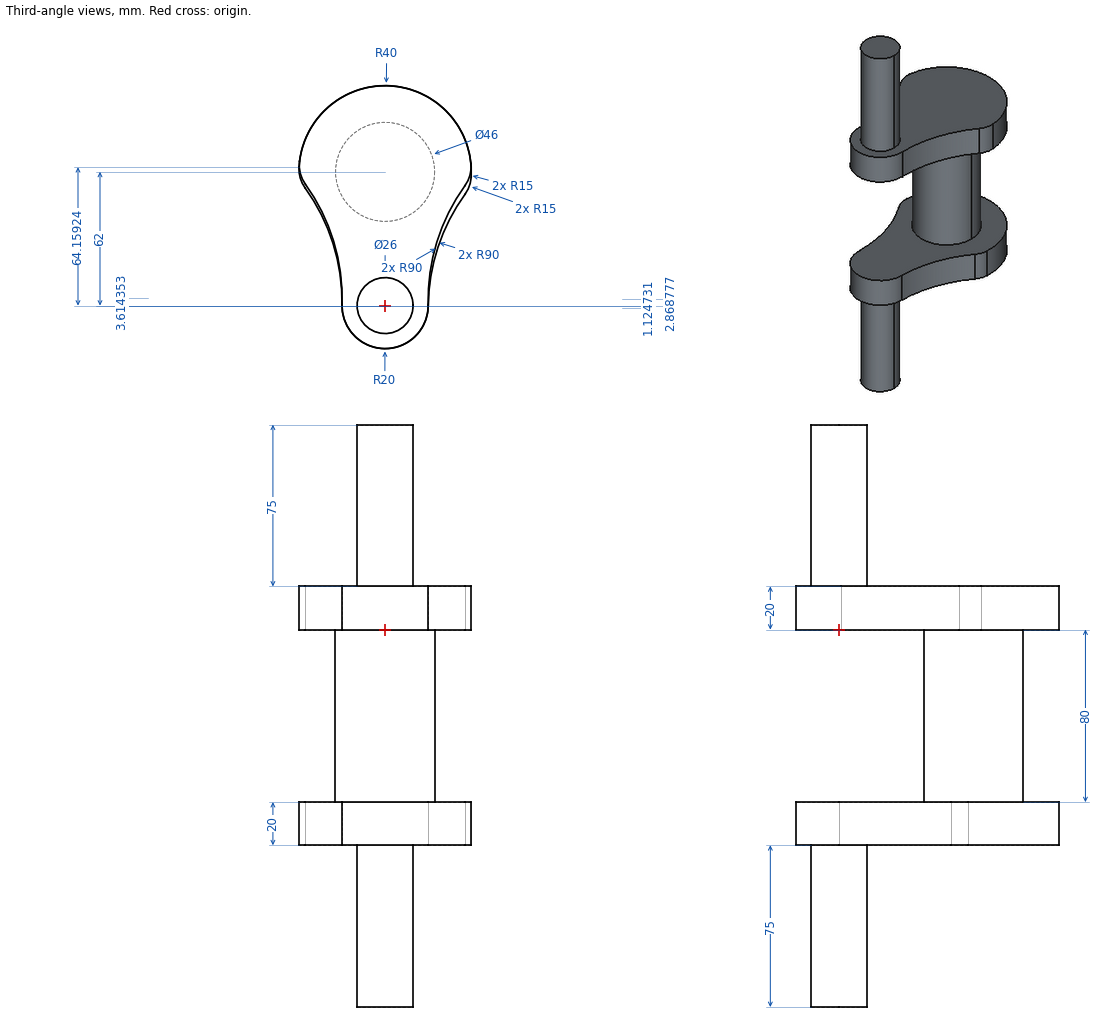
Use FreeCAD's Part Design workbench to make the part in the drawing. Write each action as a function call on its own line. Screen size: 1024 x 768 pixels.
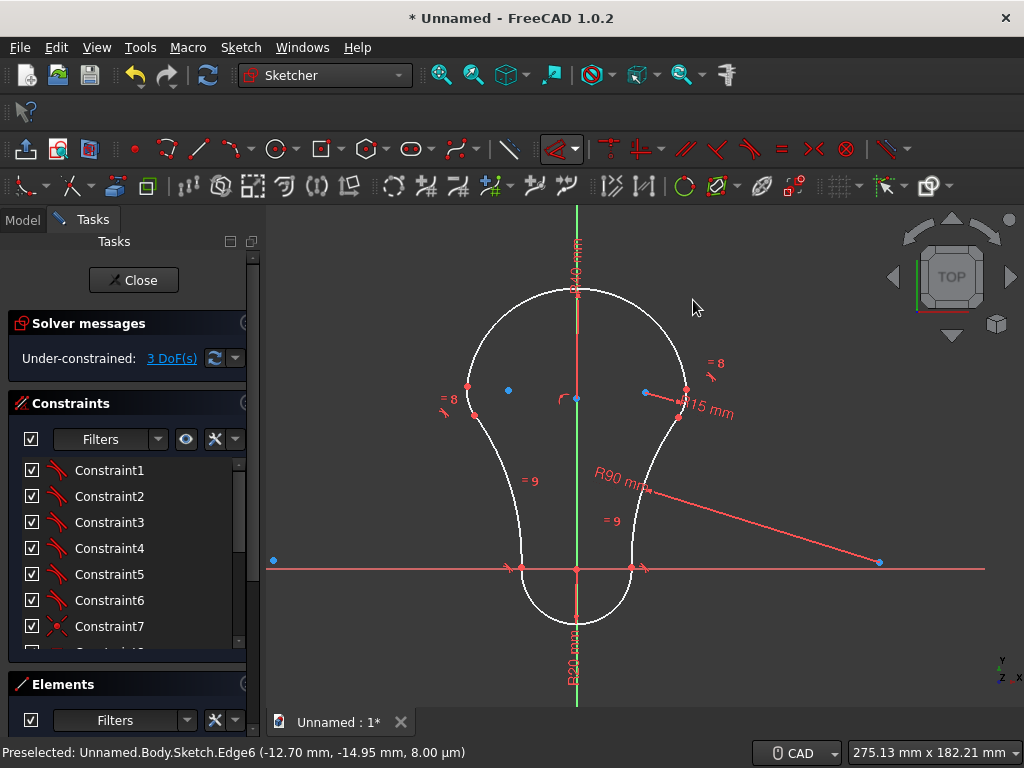
click(577, 399)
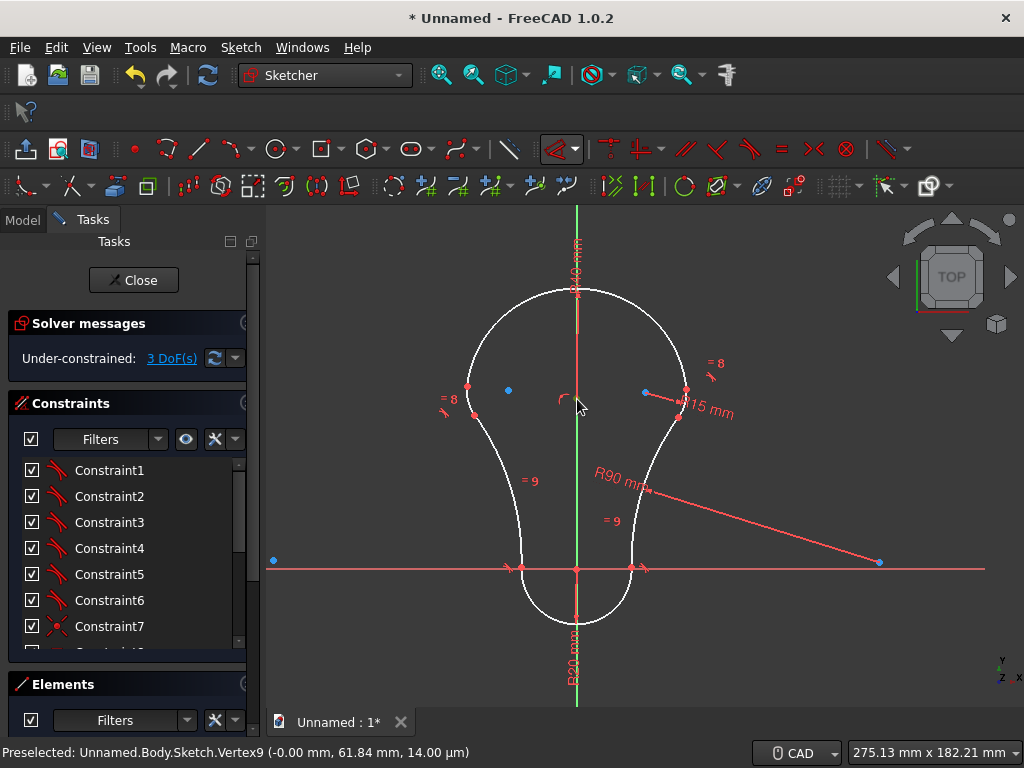
key(i)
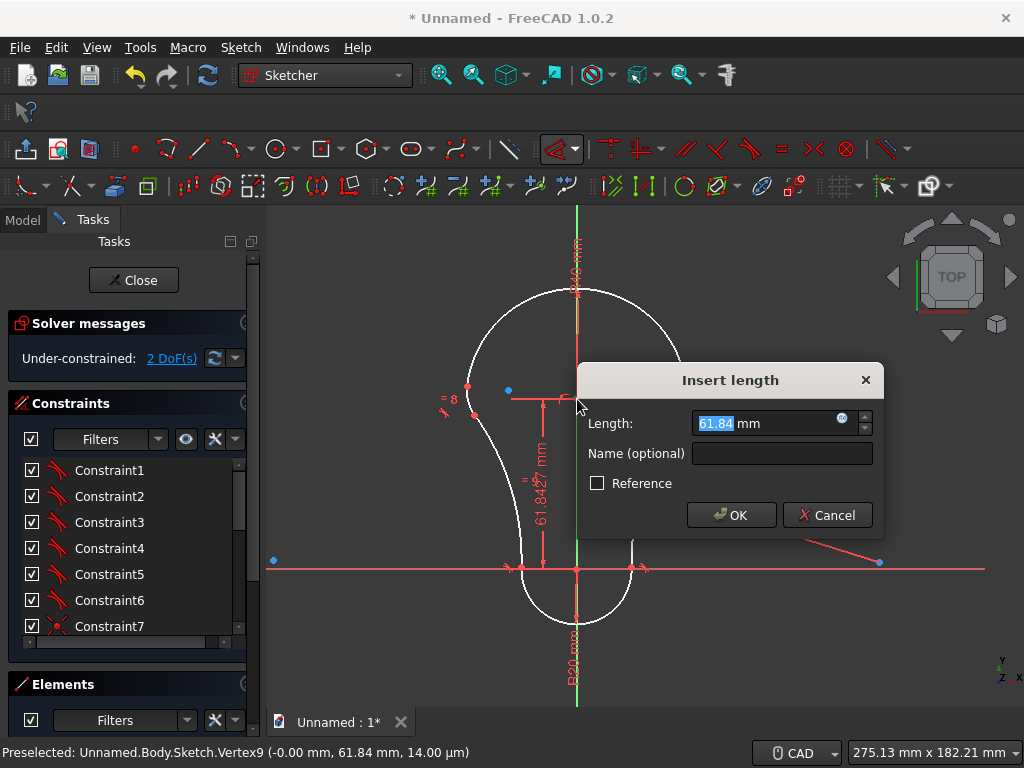
text(62)
key(Return)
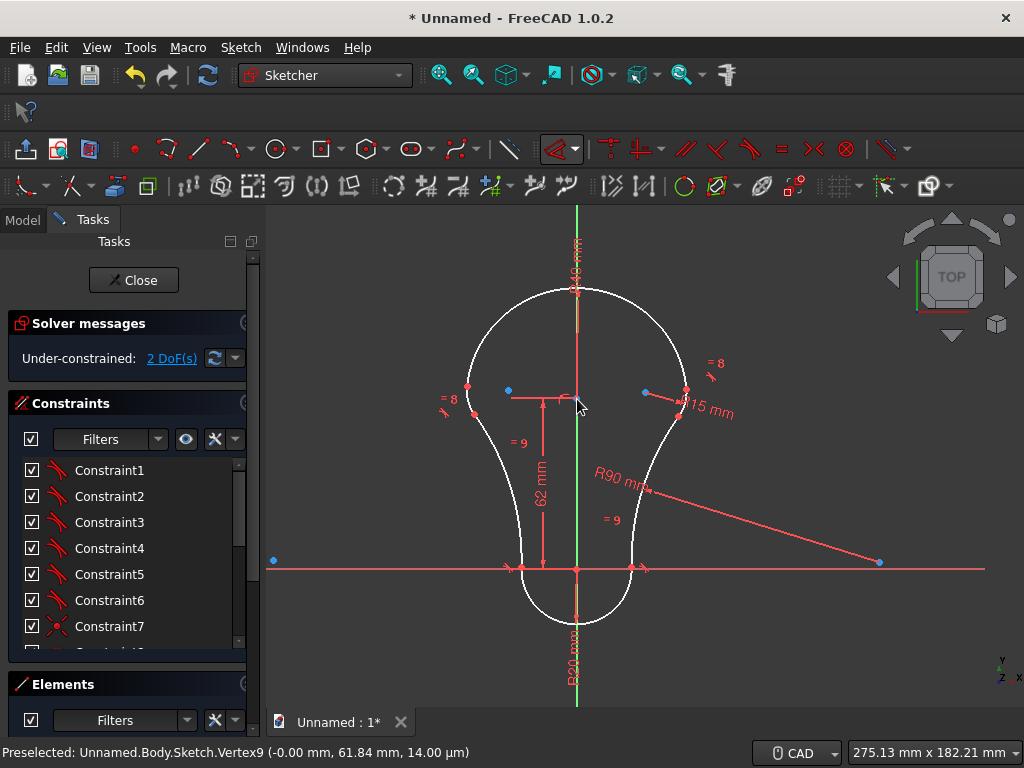
scroll(294, 455, down, 1)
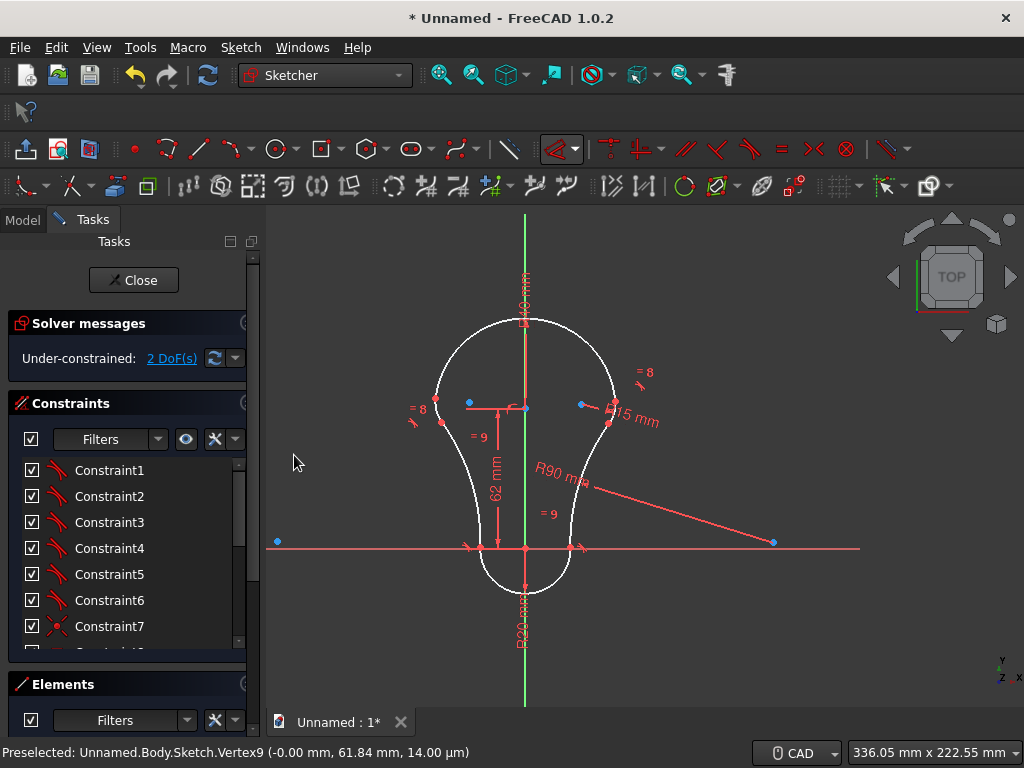
scroll(773, 543, up, 10)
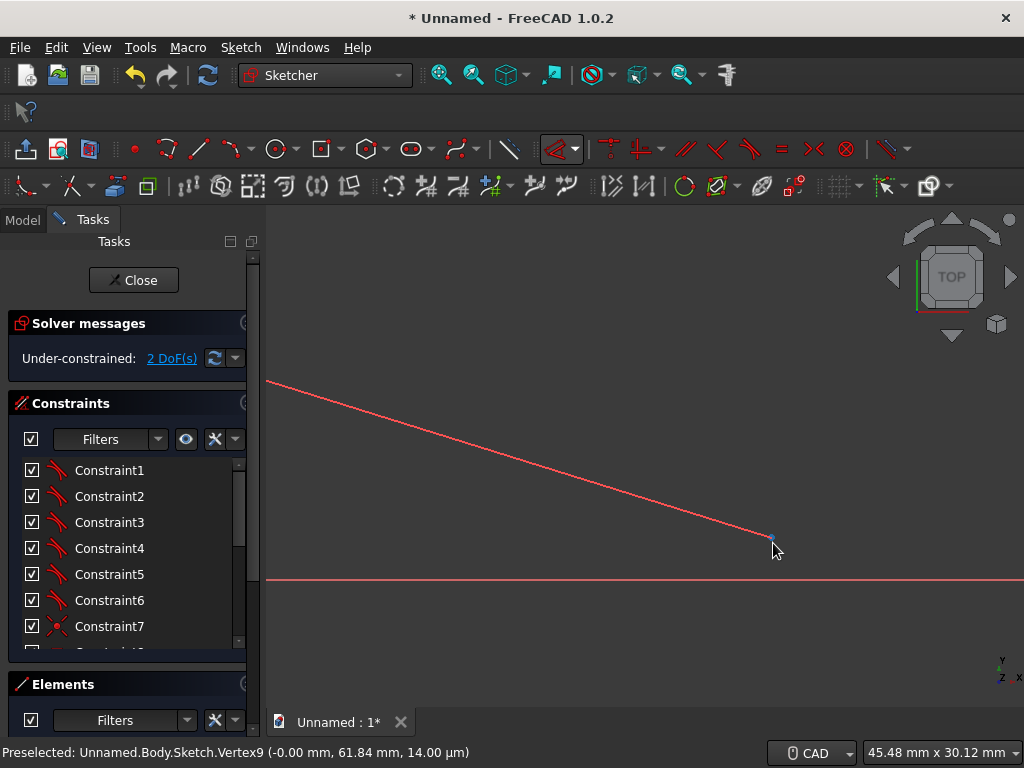
click(772, 538)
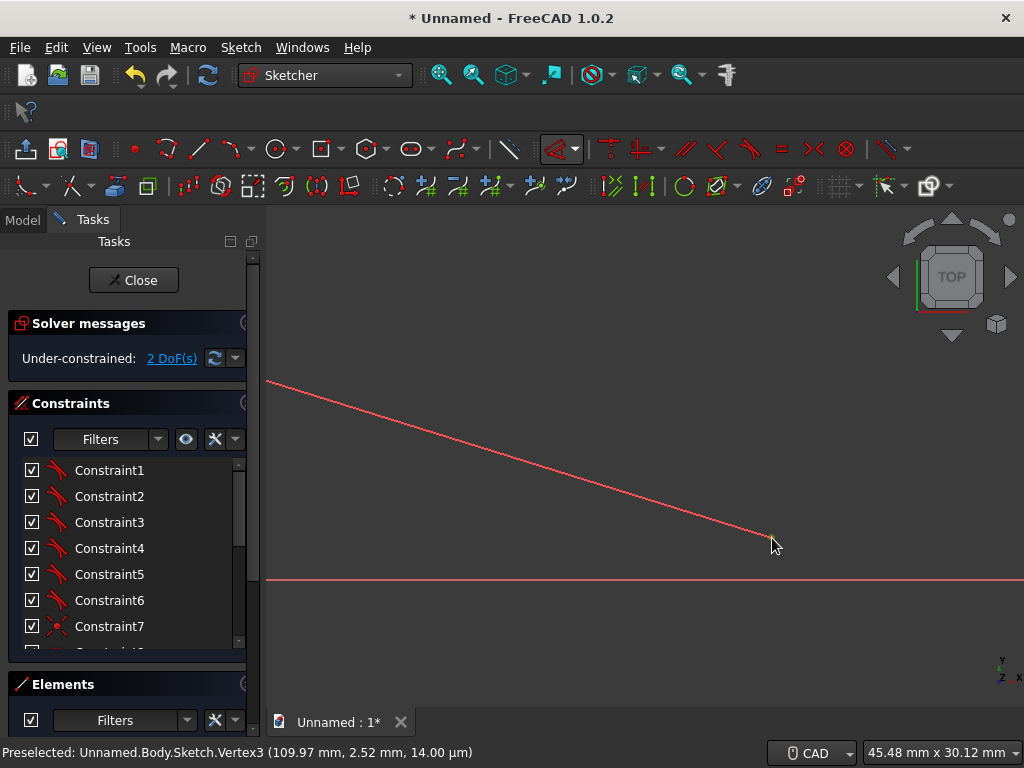
key(i)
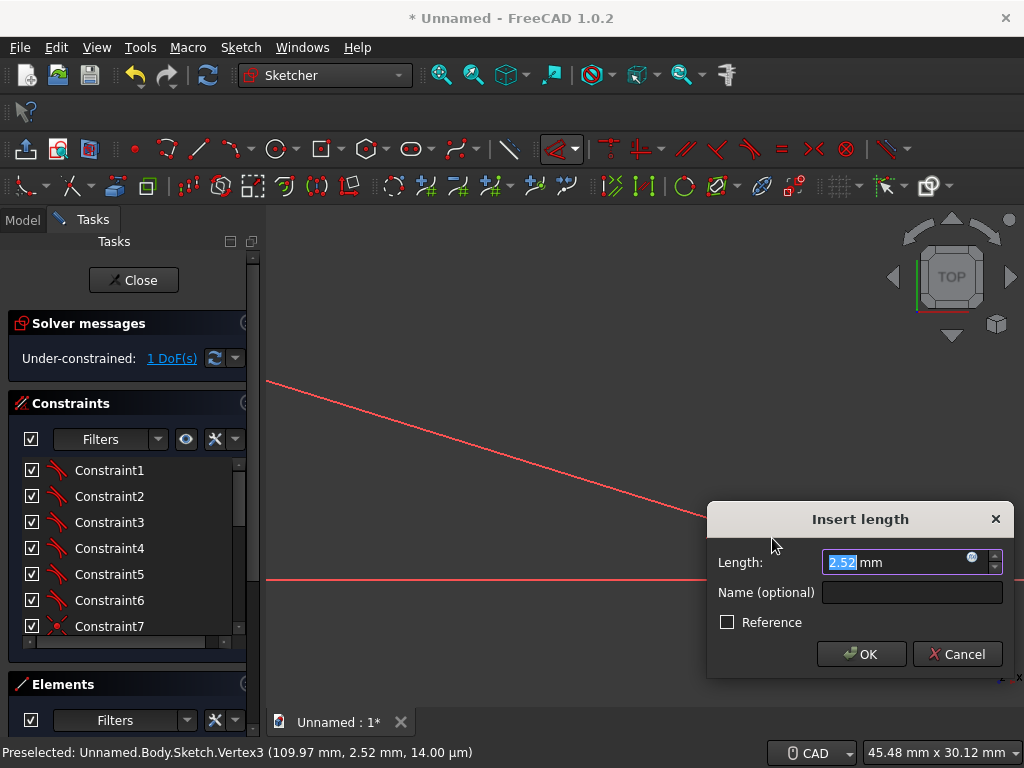
text(2.868777)
key(Return)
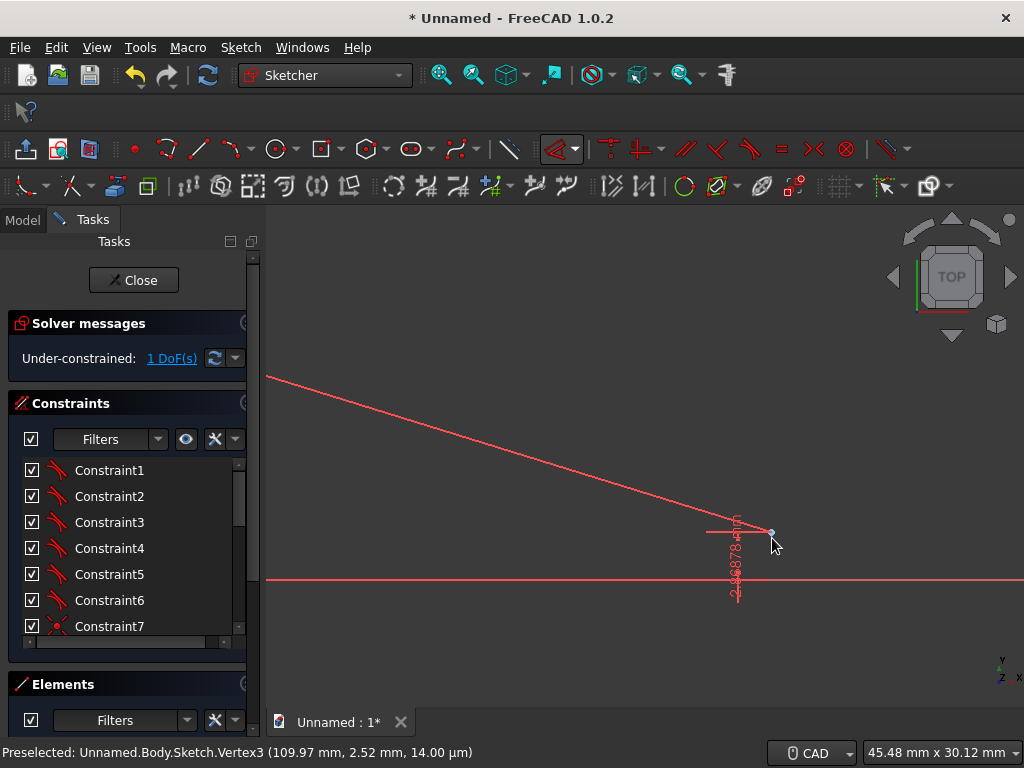
scroll(859, 567, down, 9)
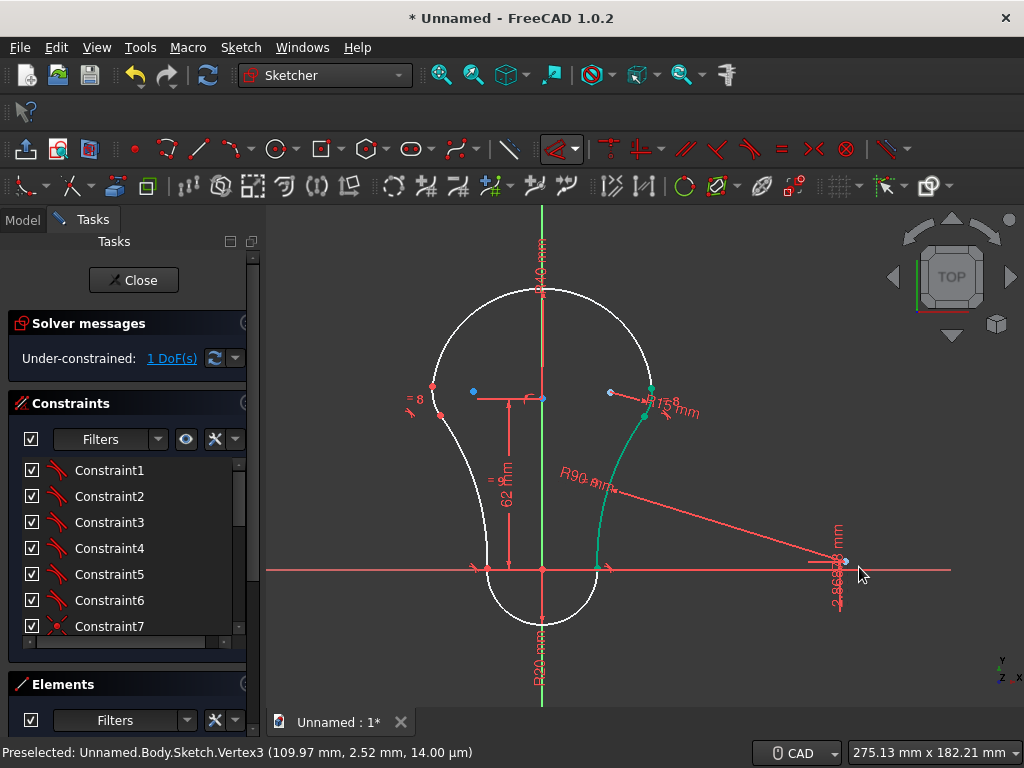
scroll(859, 452, down, 1)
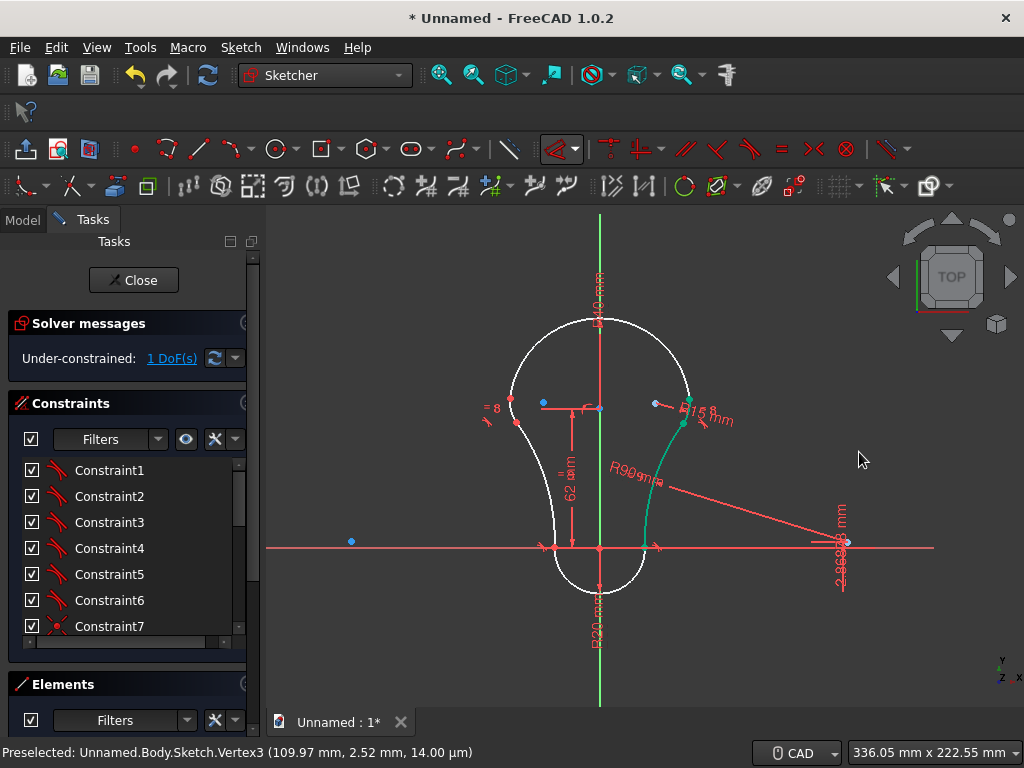
scroll(352, 541, up, 8)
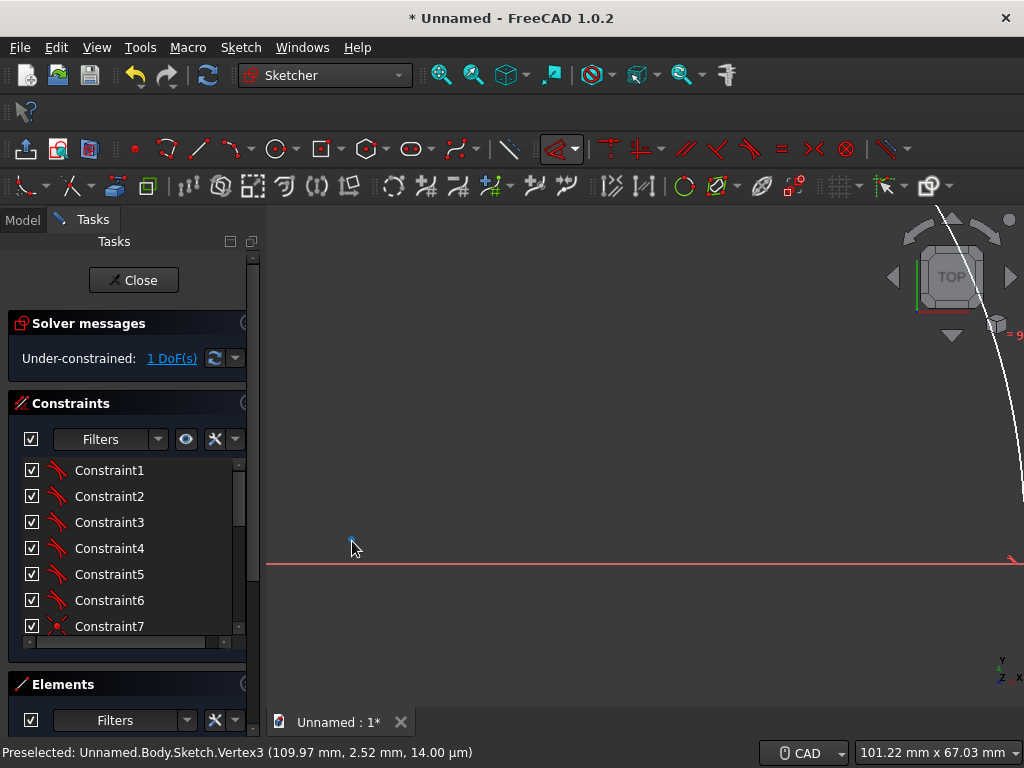
click(351, 538)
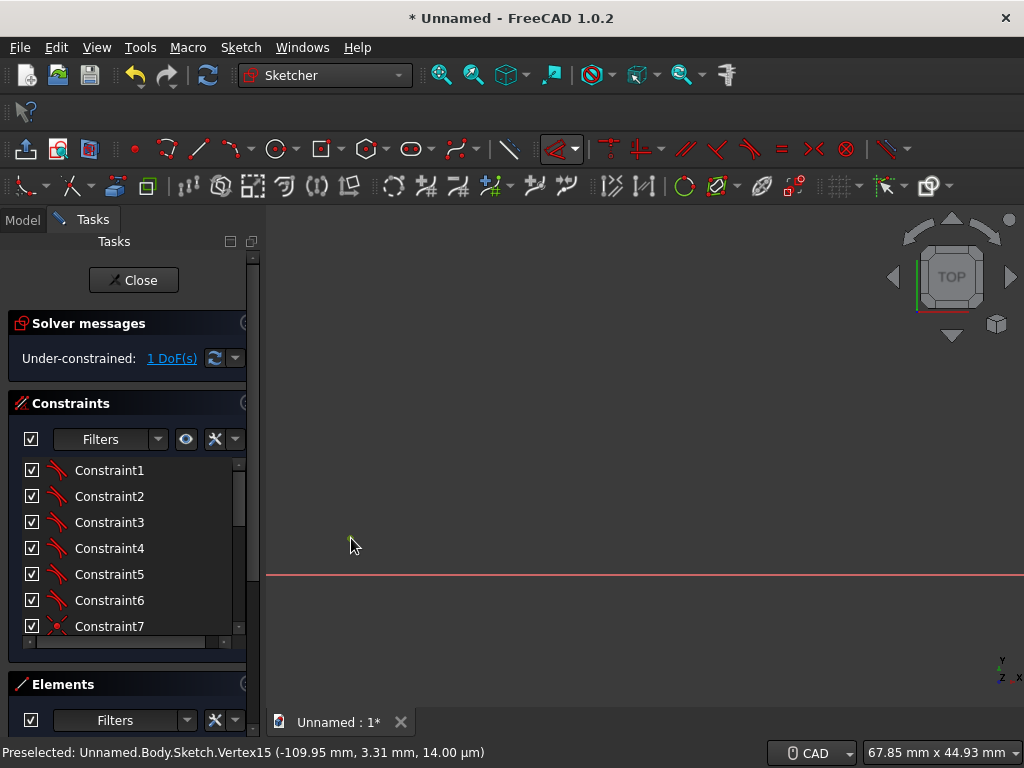
key(i)